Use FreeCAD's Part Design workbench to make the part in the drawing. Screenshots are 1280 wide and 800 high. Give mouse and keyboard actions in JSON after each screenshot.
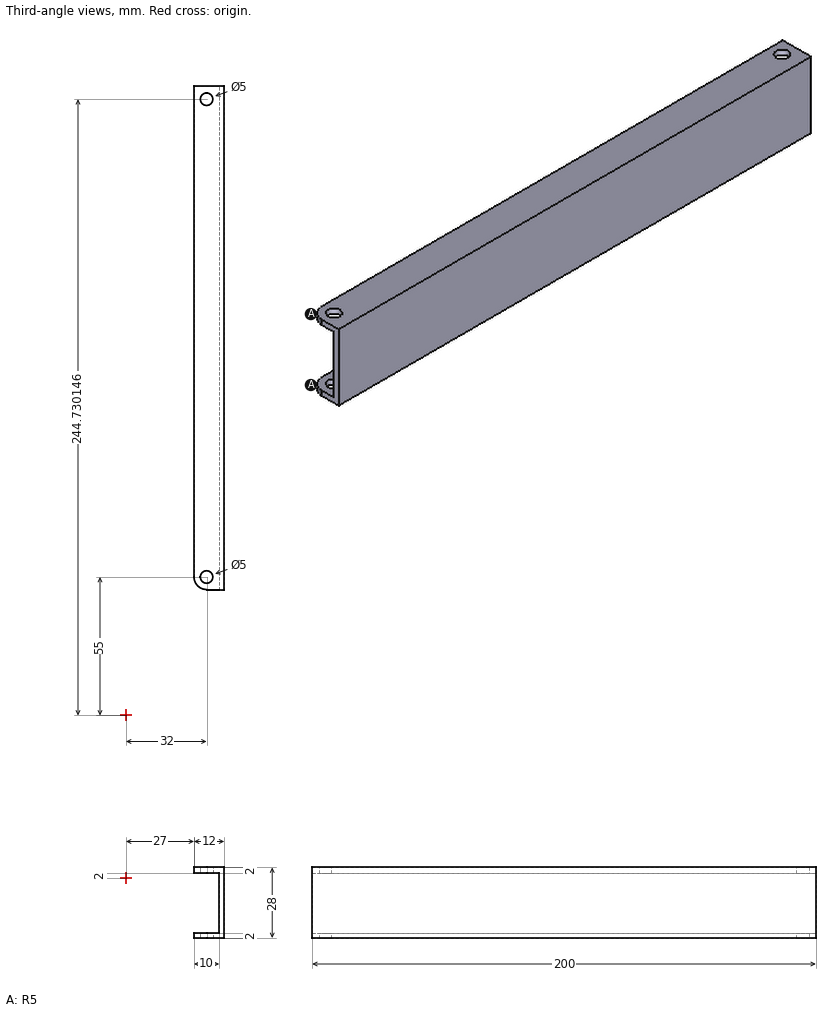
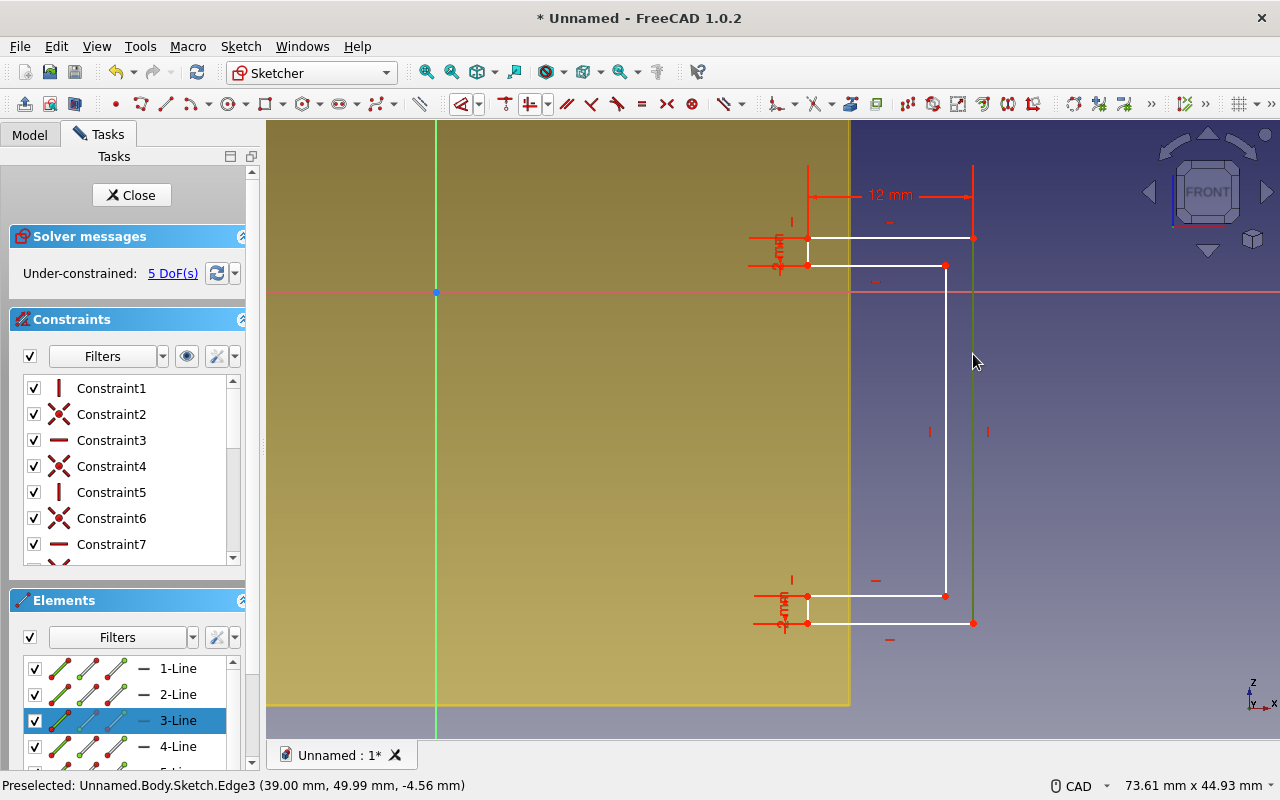
{"action": "left_click", "coordinate": [478, 104]}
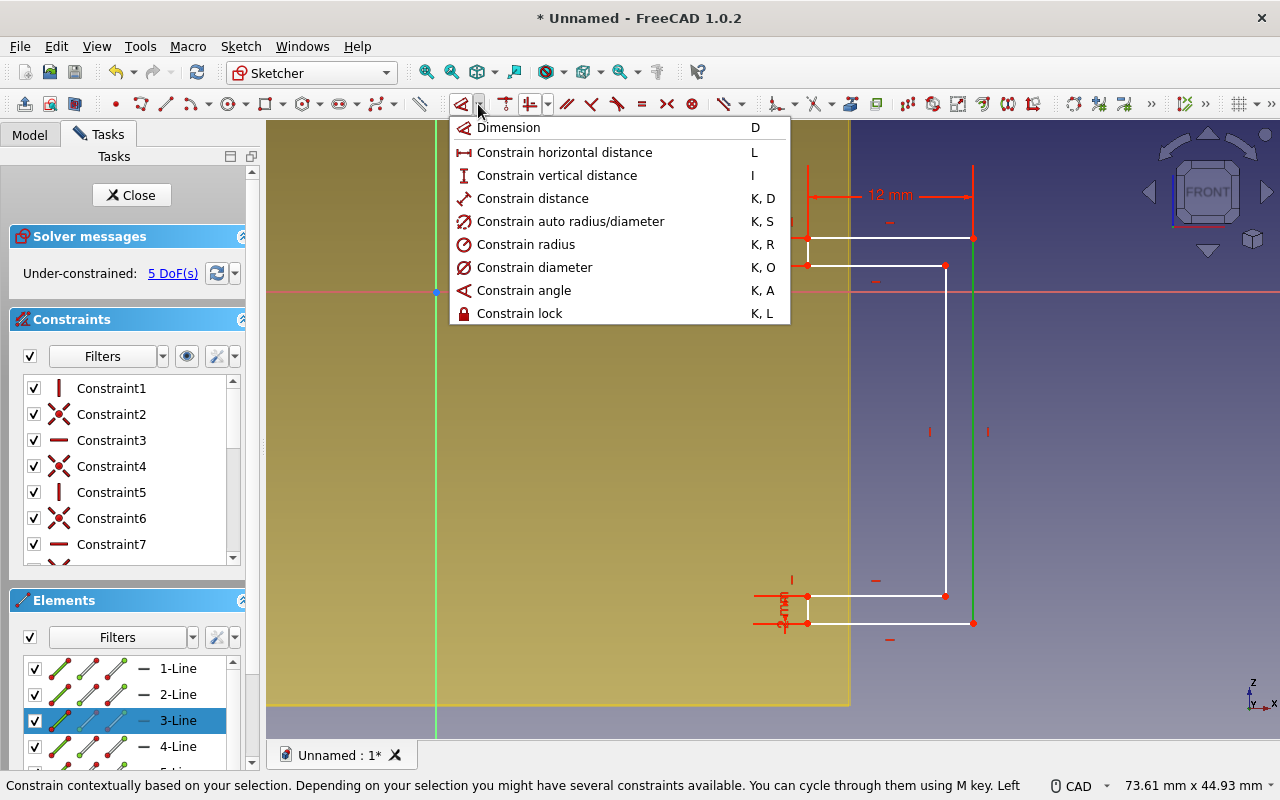
{"action": "left_click", "coordinate": [620, 176]}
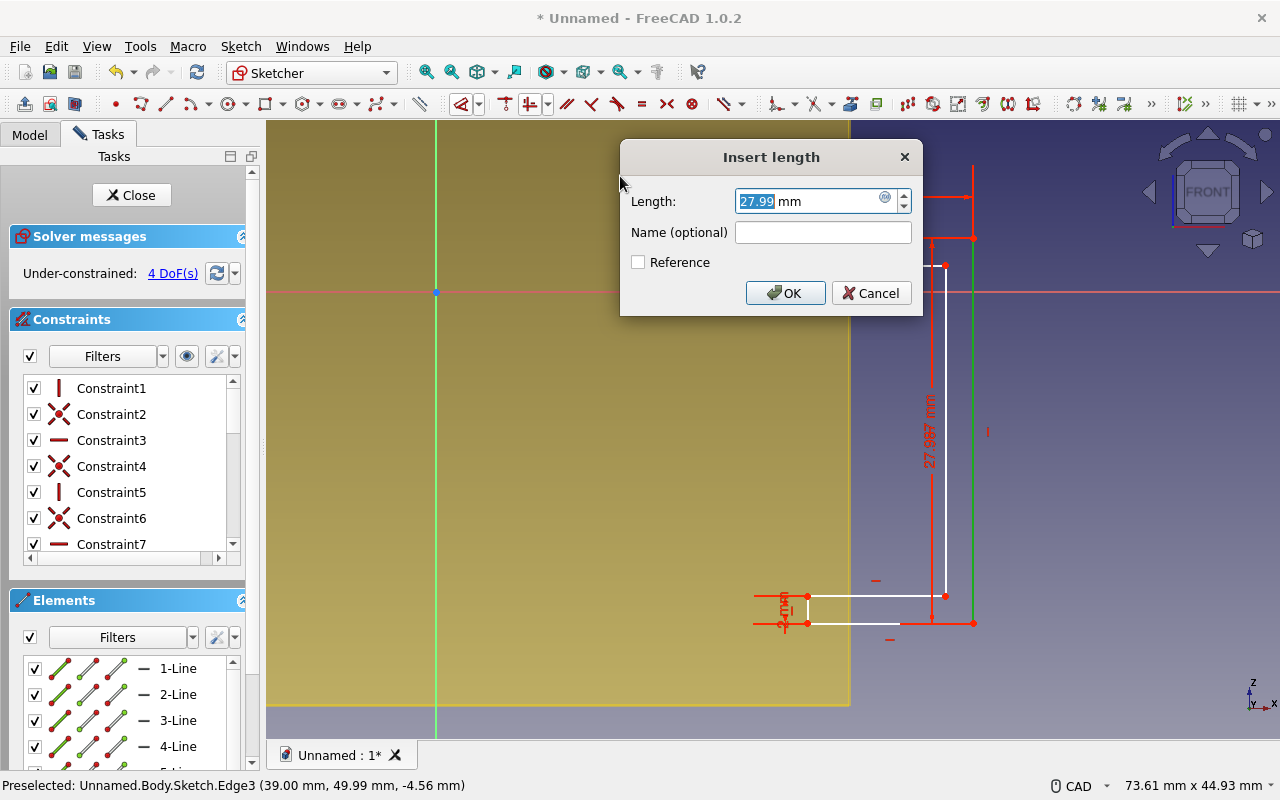
{"action": "type", "text": "28"}
{"action": "key", "text": "Return"}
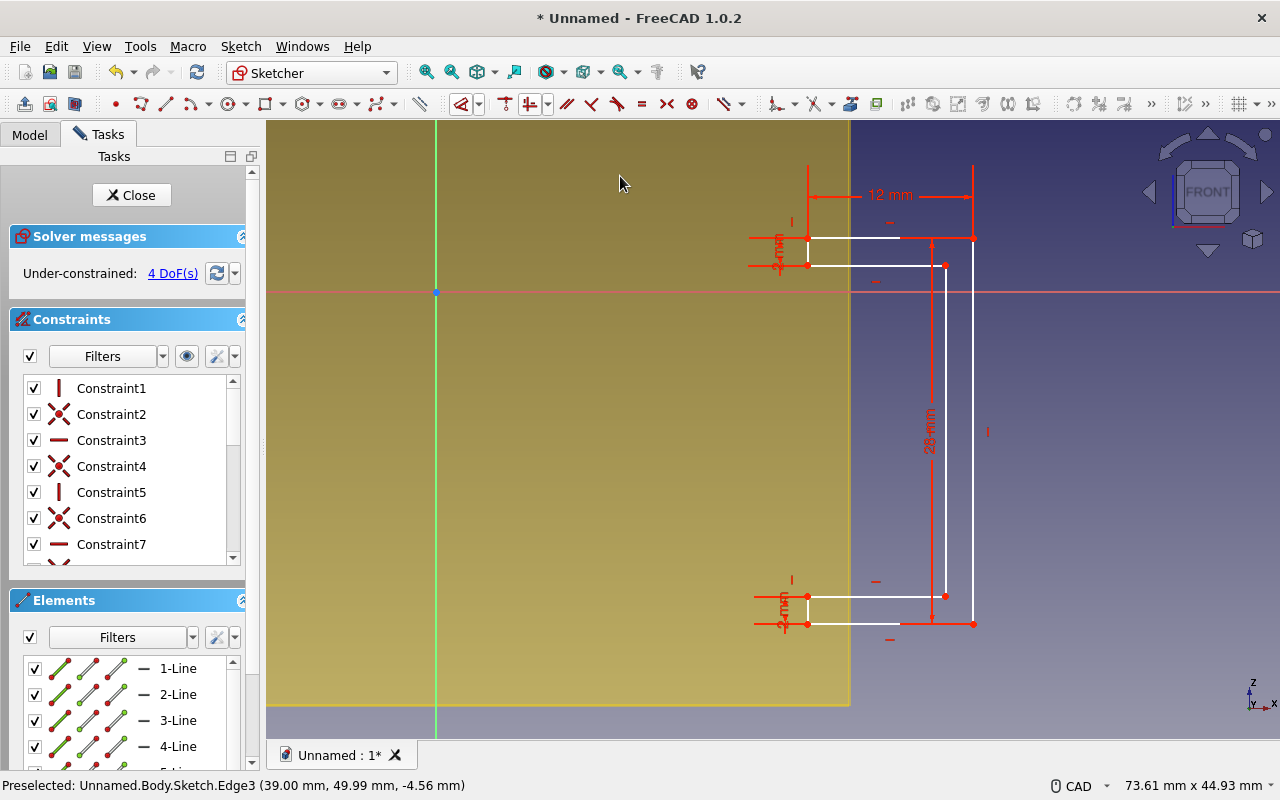
{"action": "left_click", "coordinate": [924, 624]}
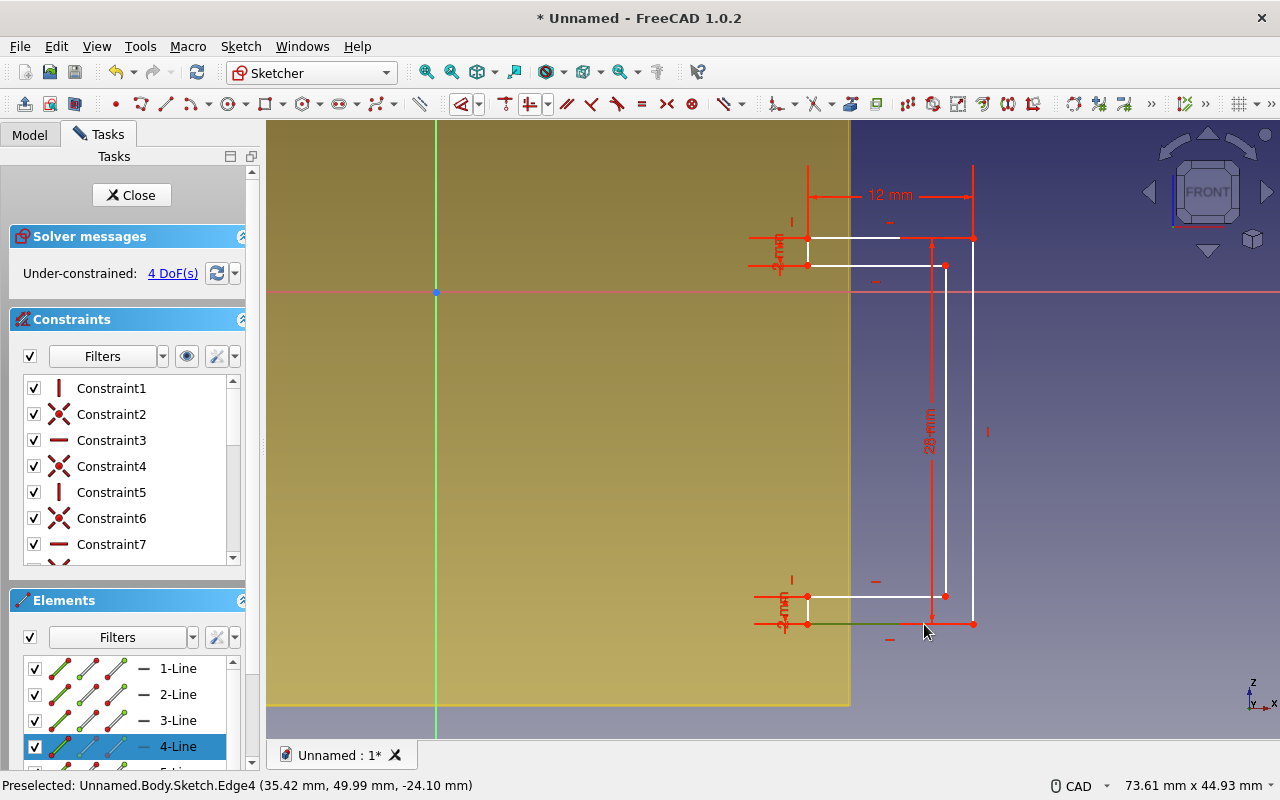
{"action": "left_click", "coordinate": [478, 104]}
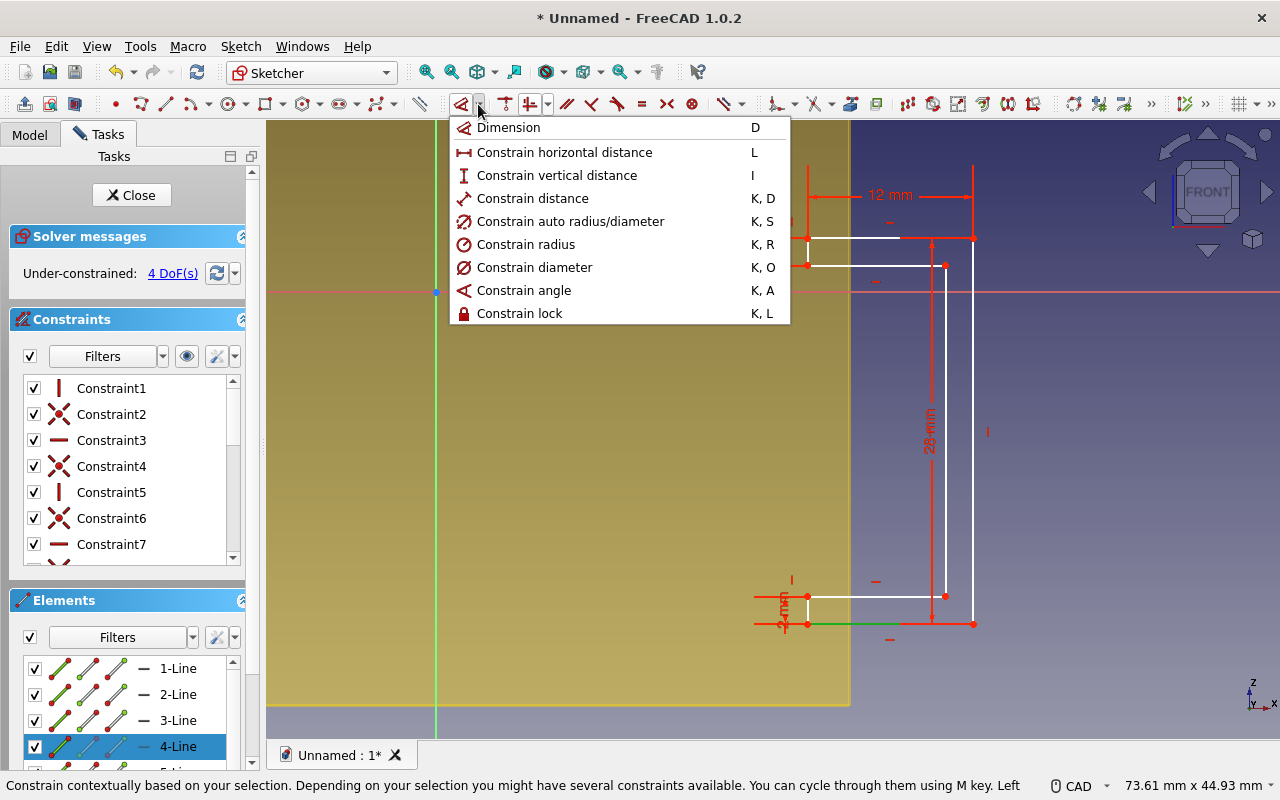
{"action": "left_click", "coordinate": [620, 152]}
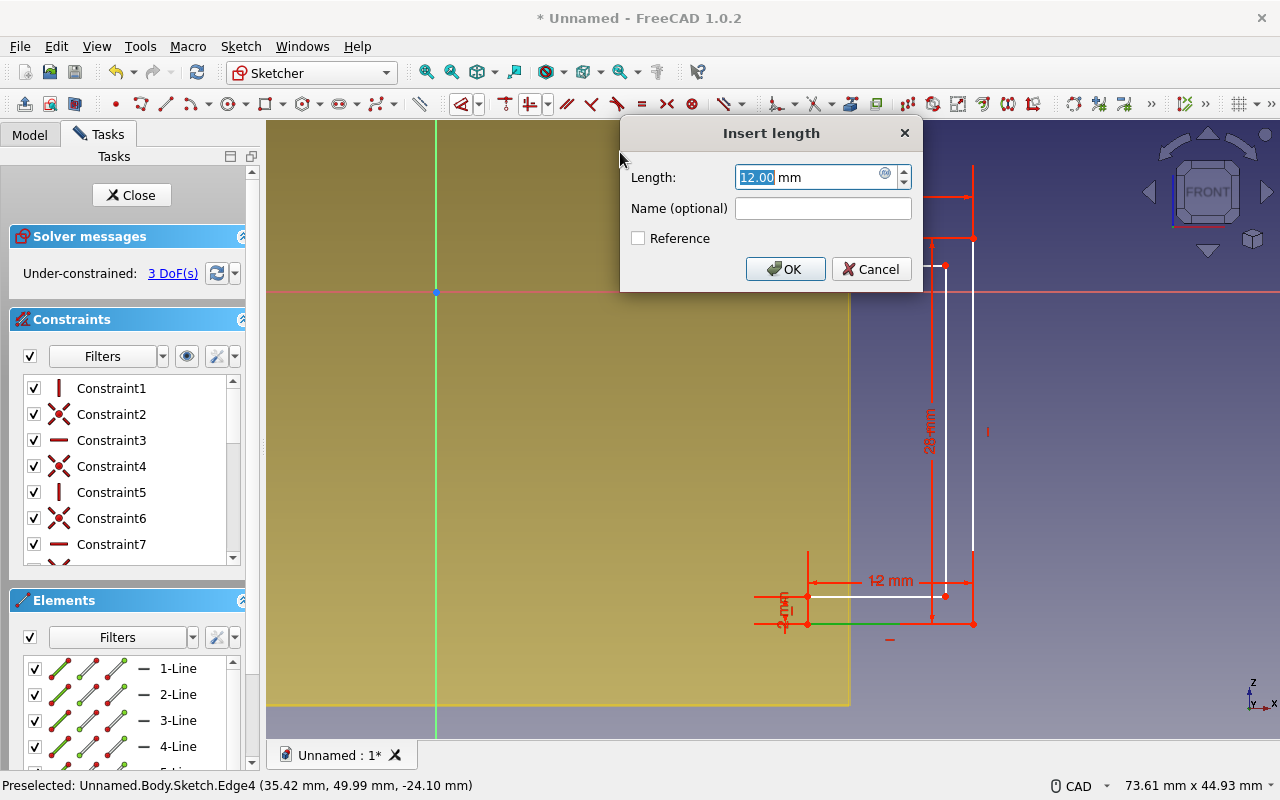
{"action": "type", "text": "12"}
{"action": "key", "text": "Return"}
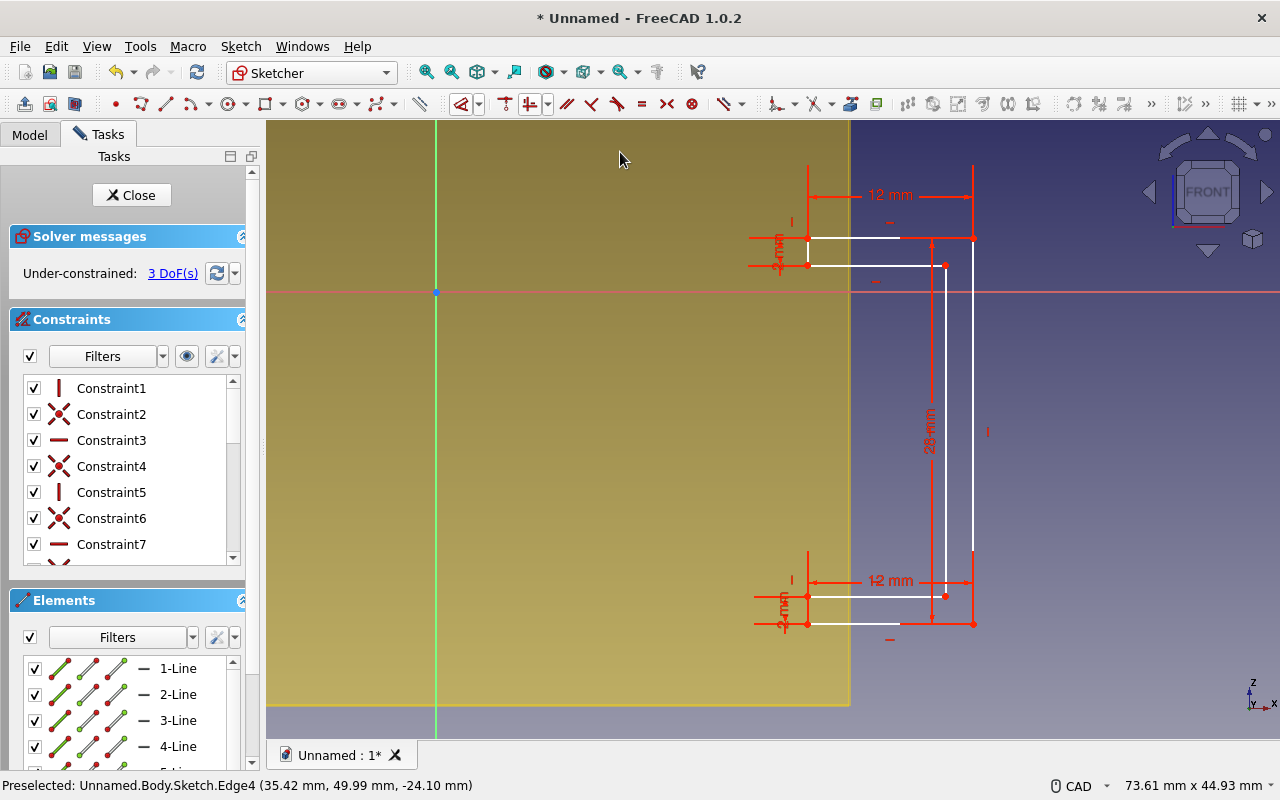
{"action": "left_click", "coordinate": [849, 597]}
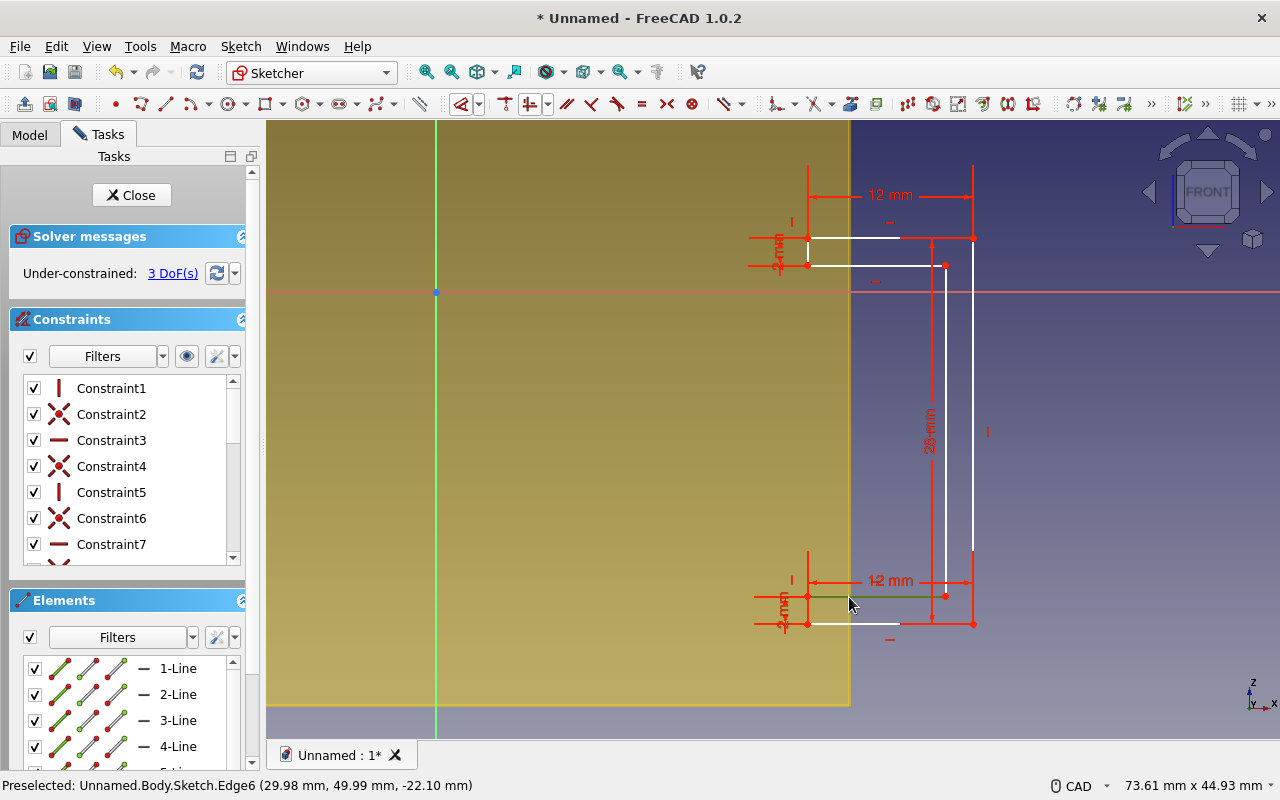
{"action": "left_click", "coordinate": [478, 104]}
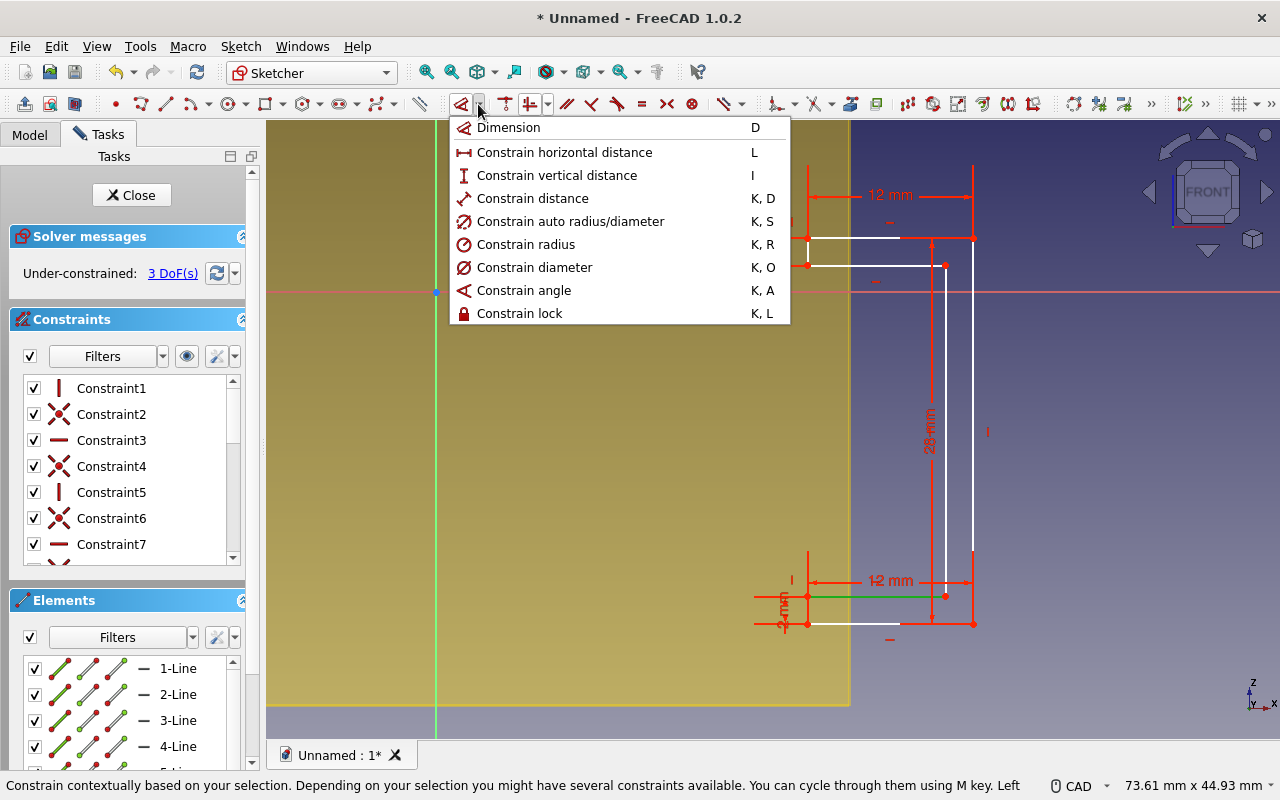
{"action": "left_click", "coordinate": [620, 152]}